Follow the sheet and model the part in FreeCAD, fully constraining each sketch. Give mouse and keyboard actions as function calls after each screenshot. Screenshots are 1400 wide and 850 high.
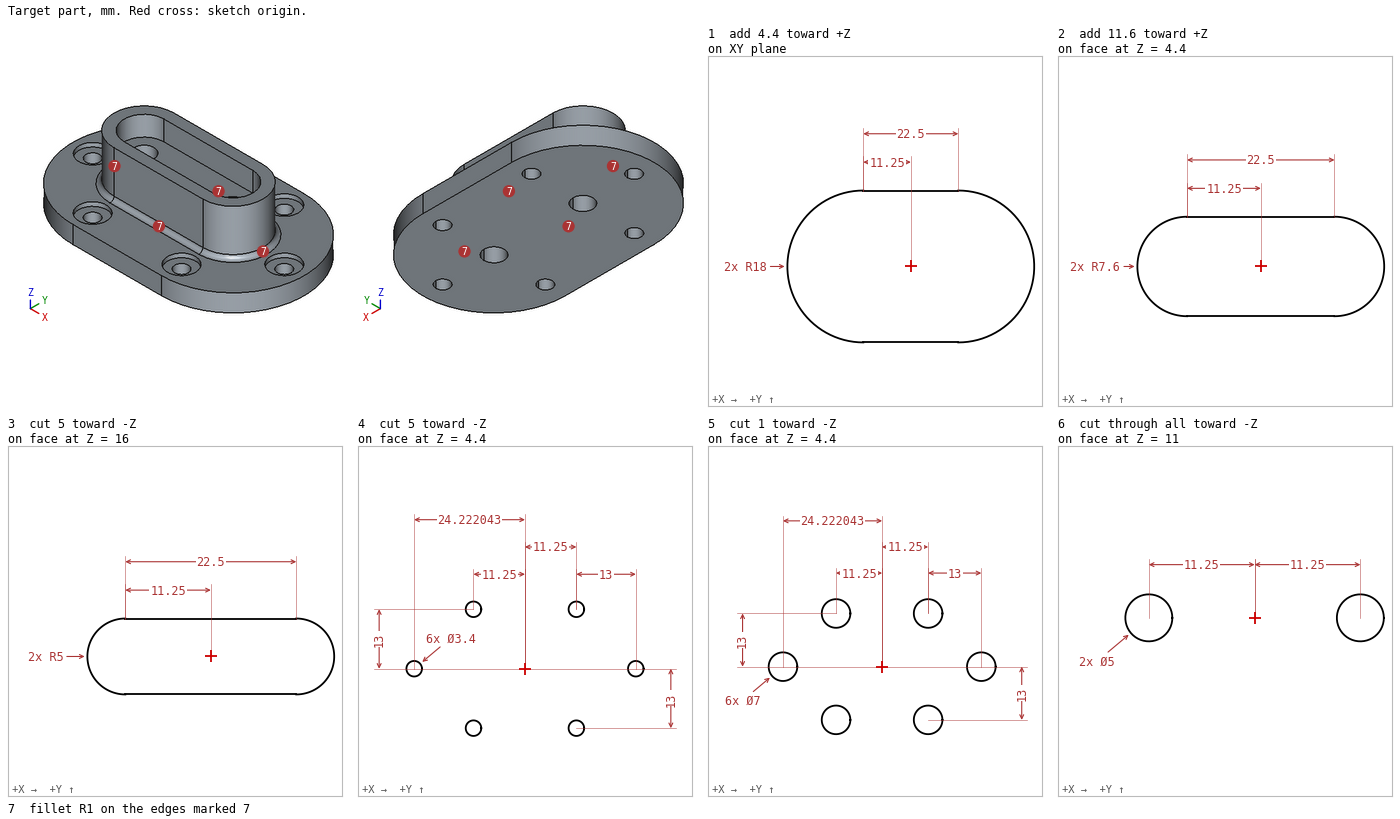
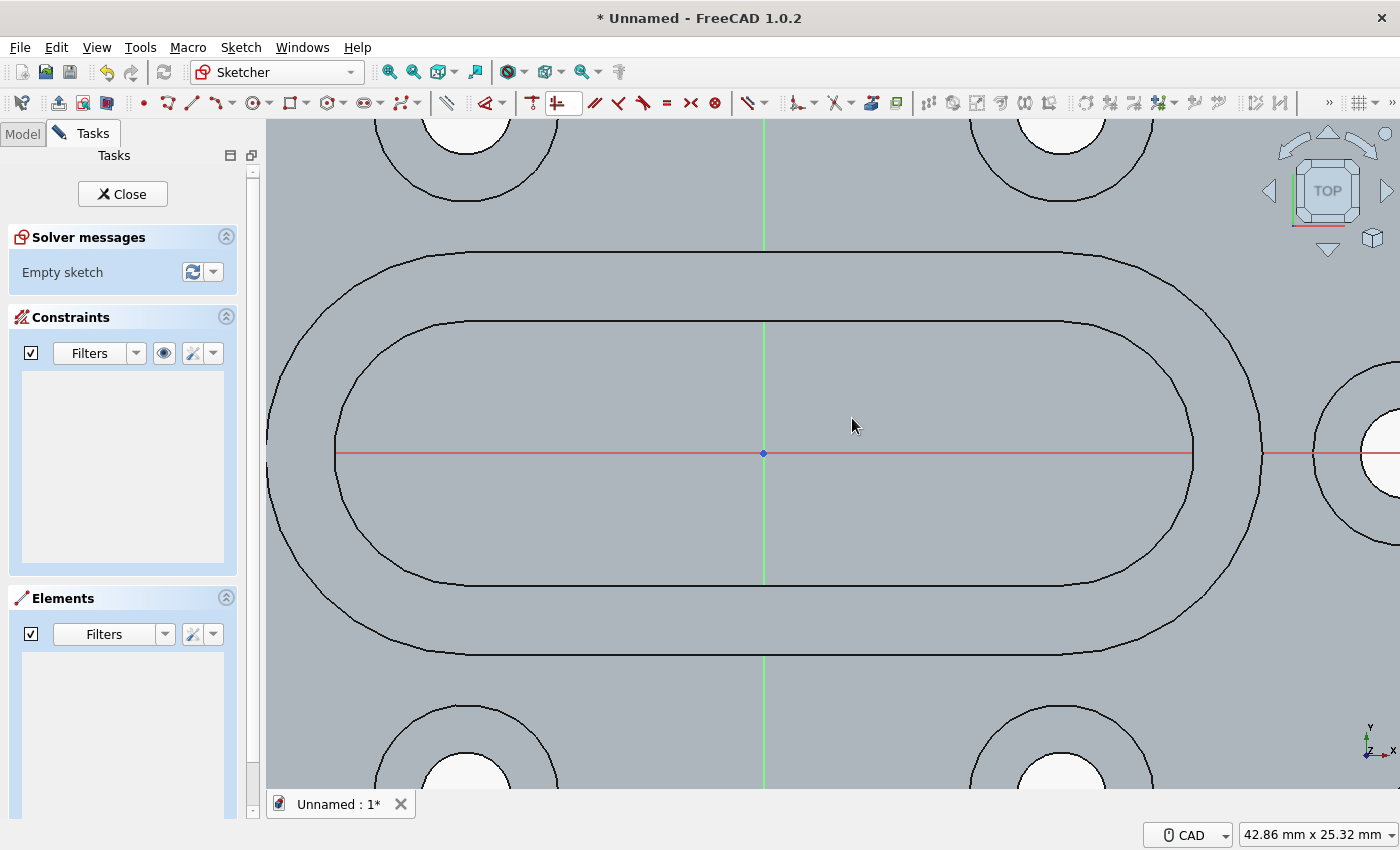
click(254, 104)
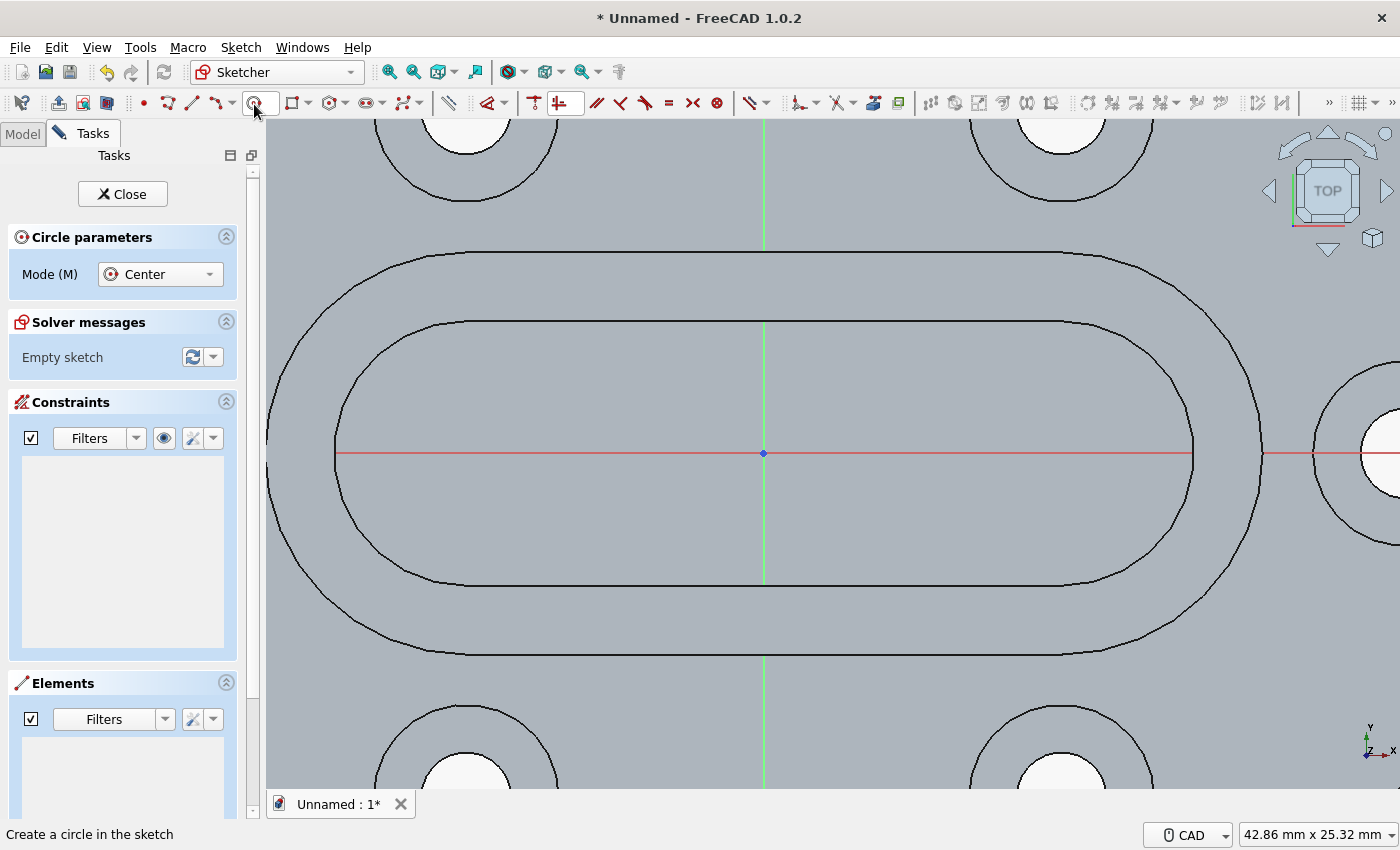
click(466, 453)
move(513, 407)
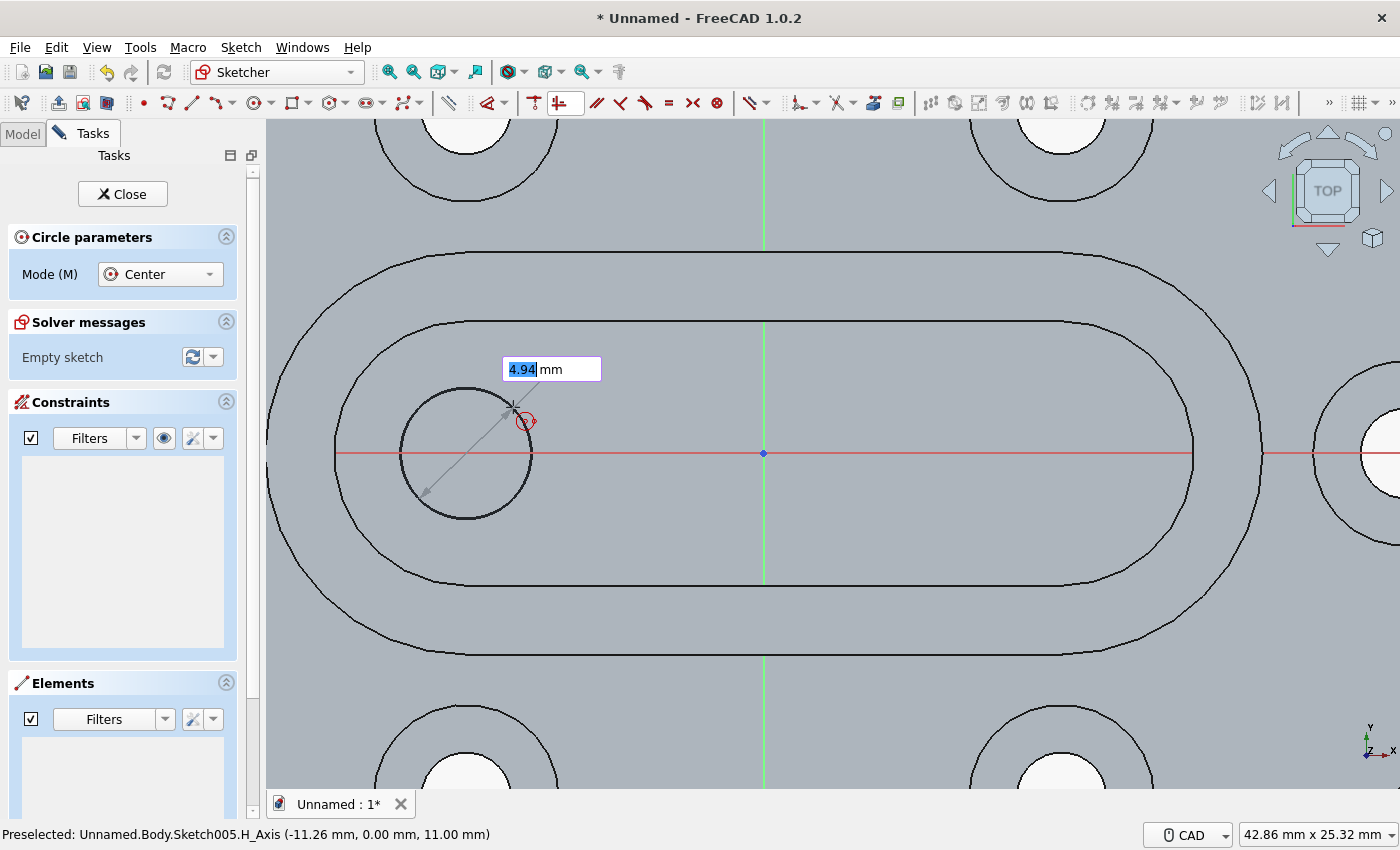
text(5)
key(Return)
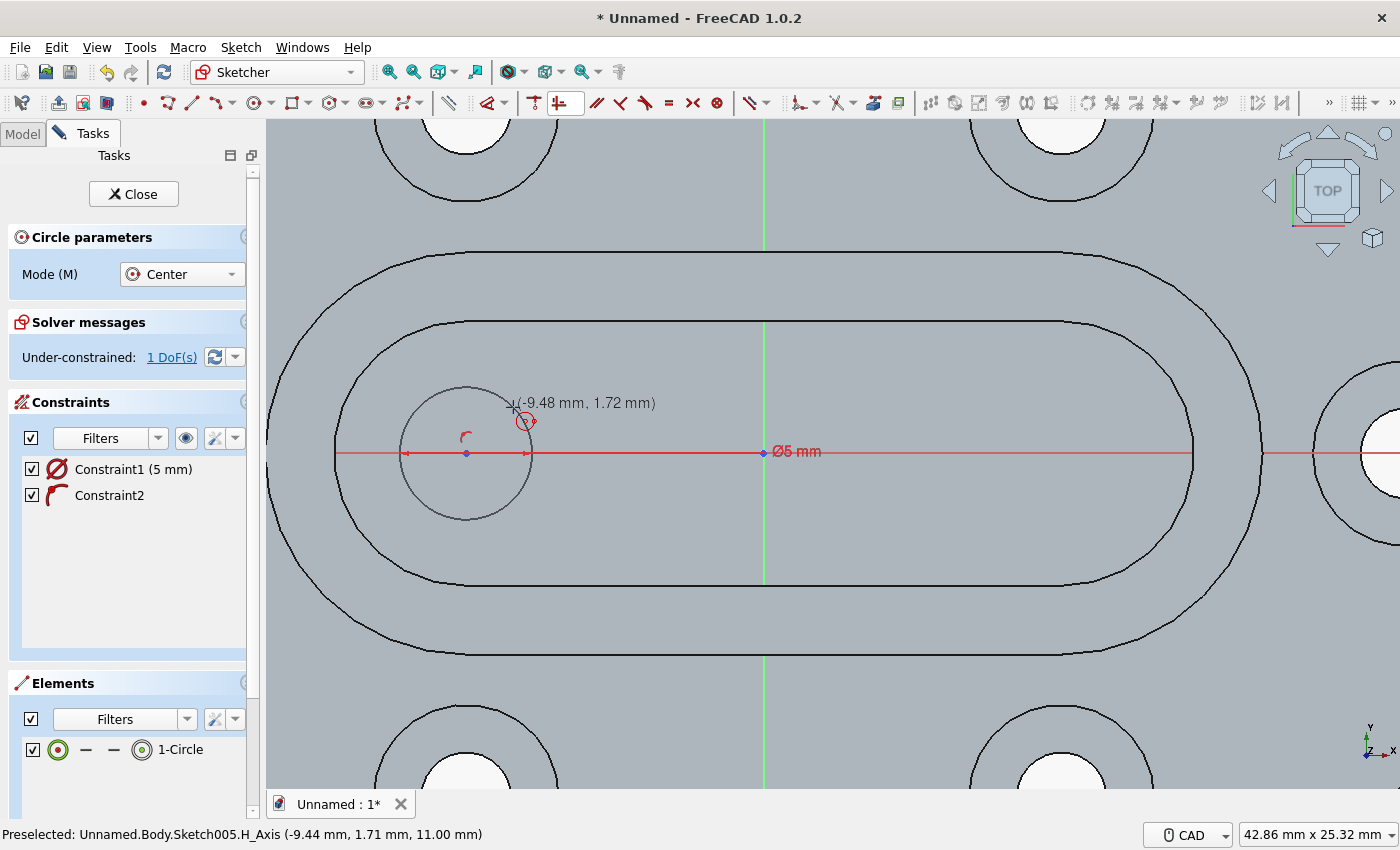
click(1062, 453)
move(1108, 407)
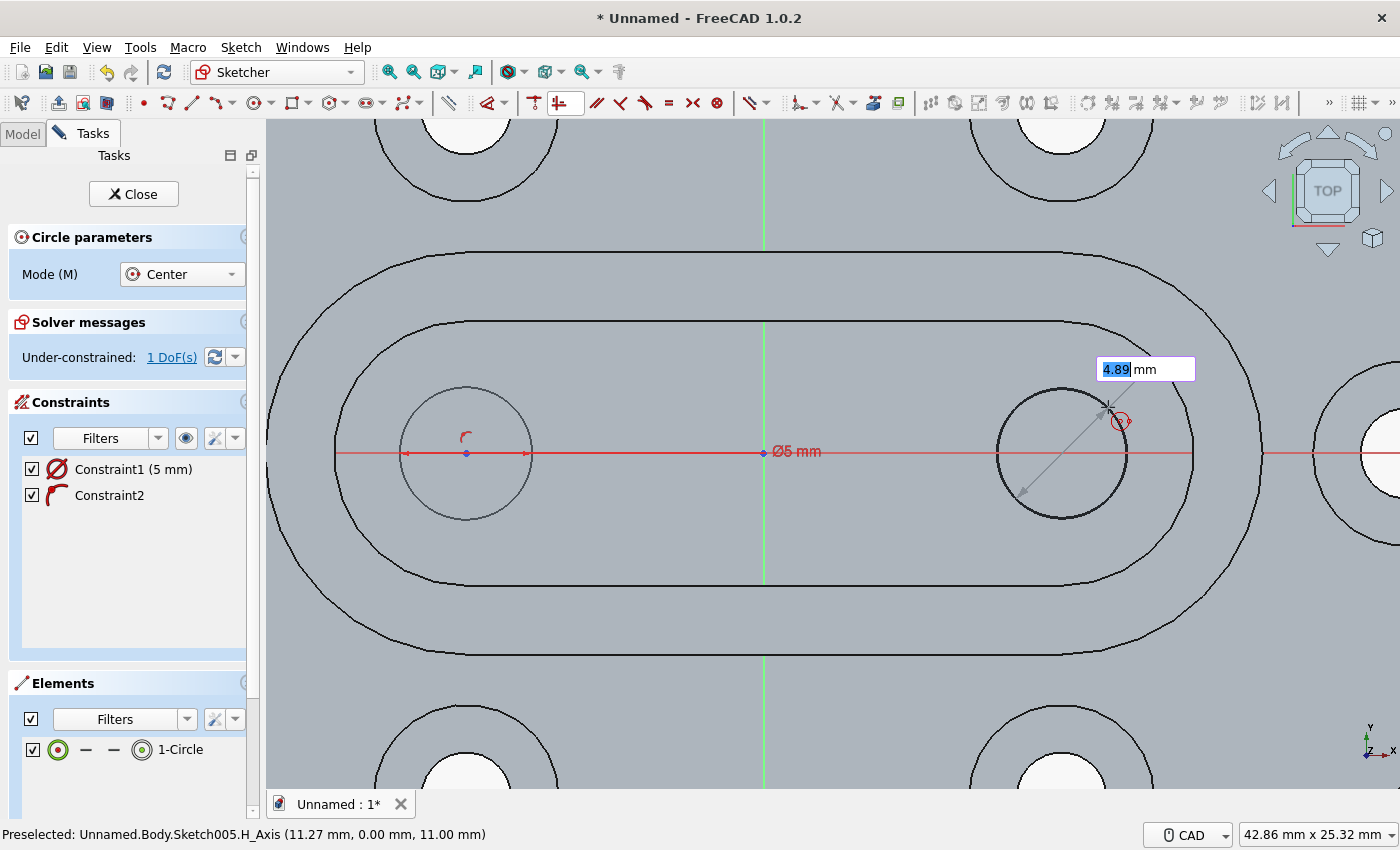
text(5)
key(Return)
key(Escape)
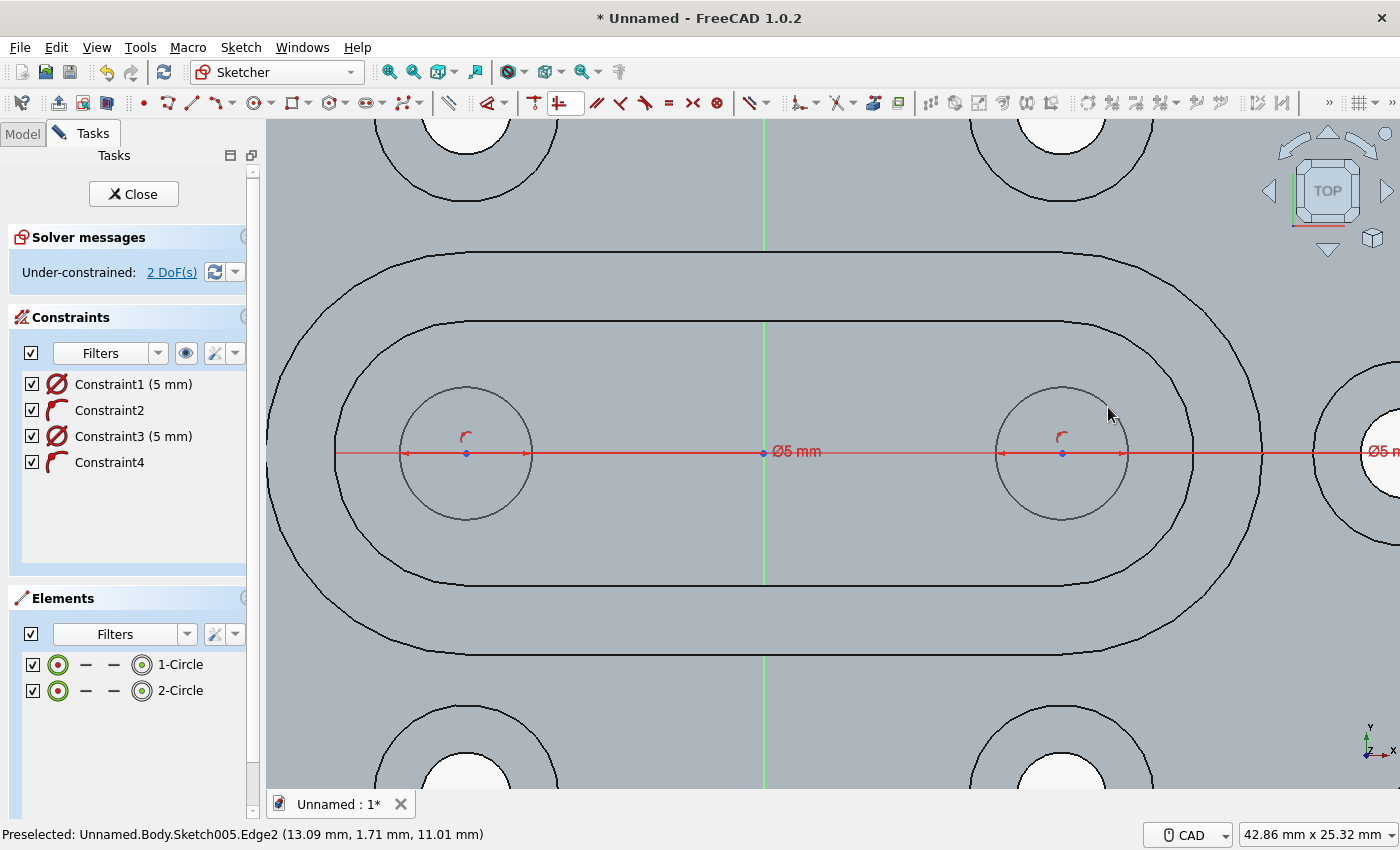
click(488, 104)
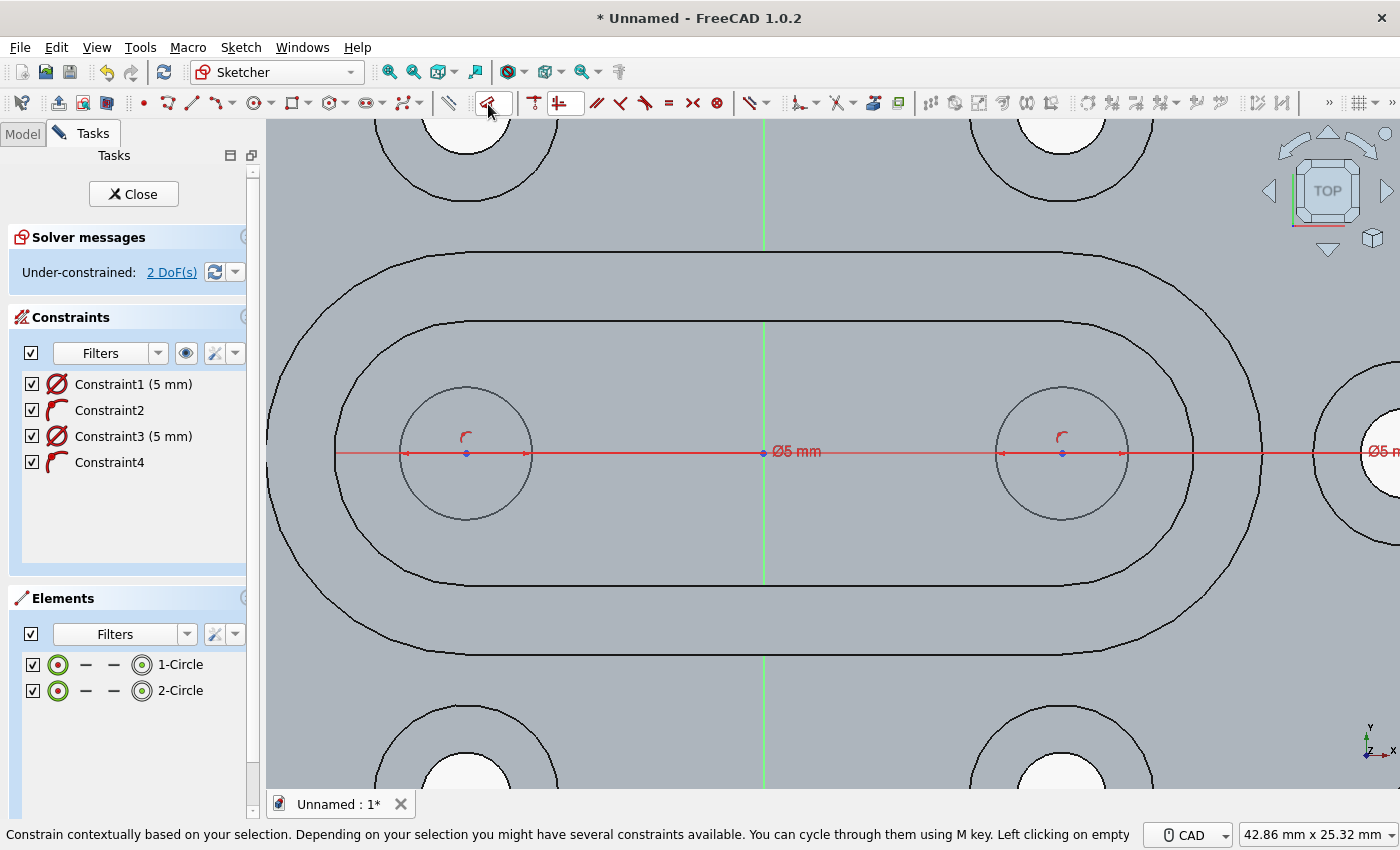
click(466, 453)
click(615, 487)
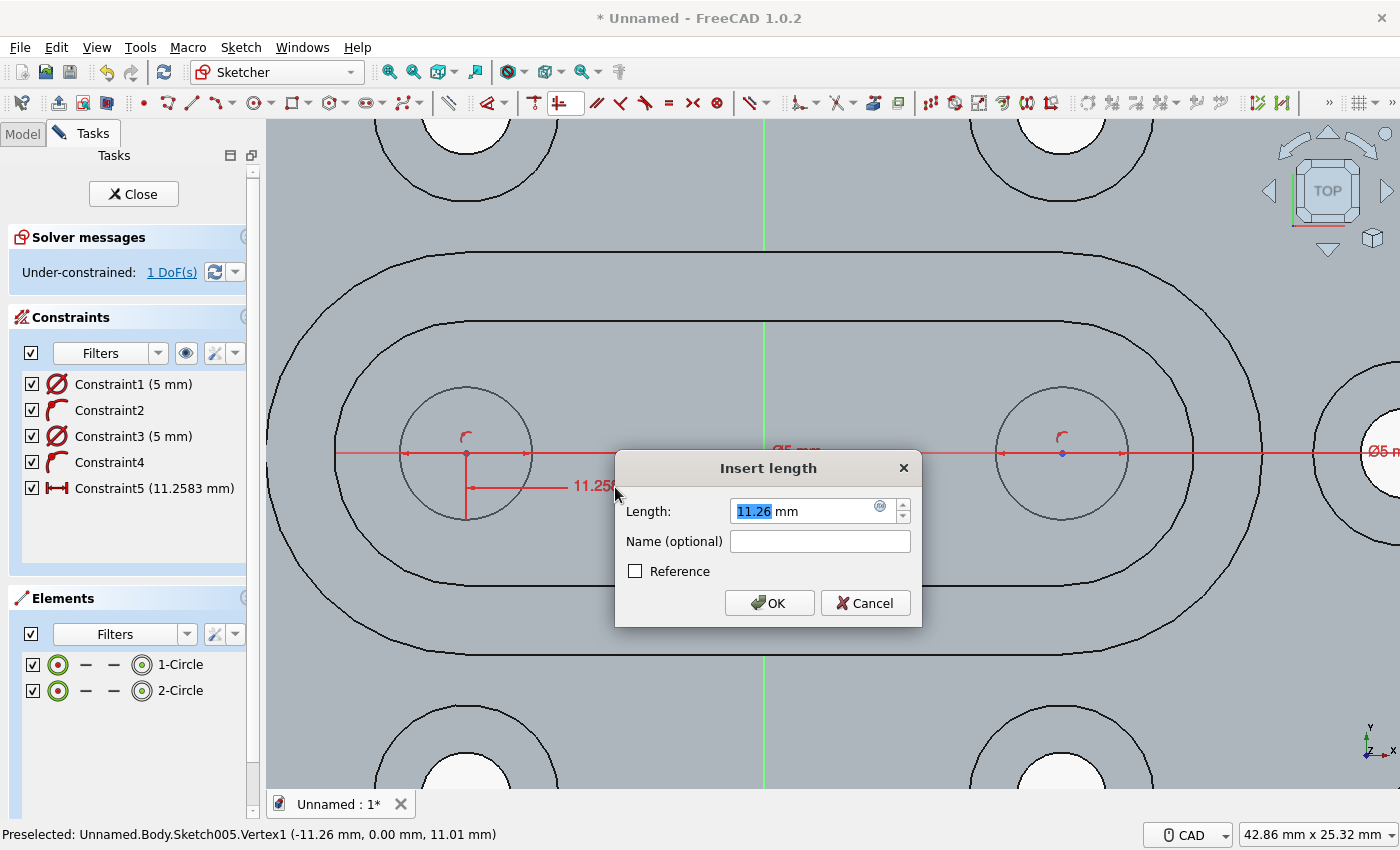
text(11.25)
key(Return)